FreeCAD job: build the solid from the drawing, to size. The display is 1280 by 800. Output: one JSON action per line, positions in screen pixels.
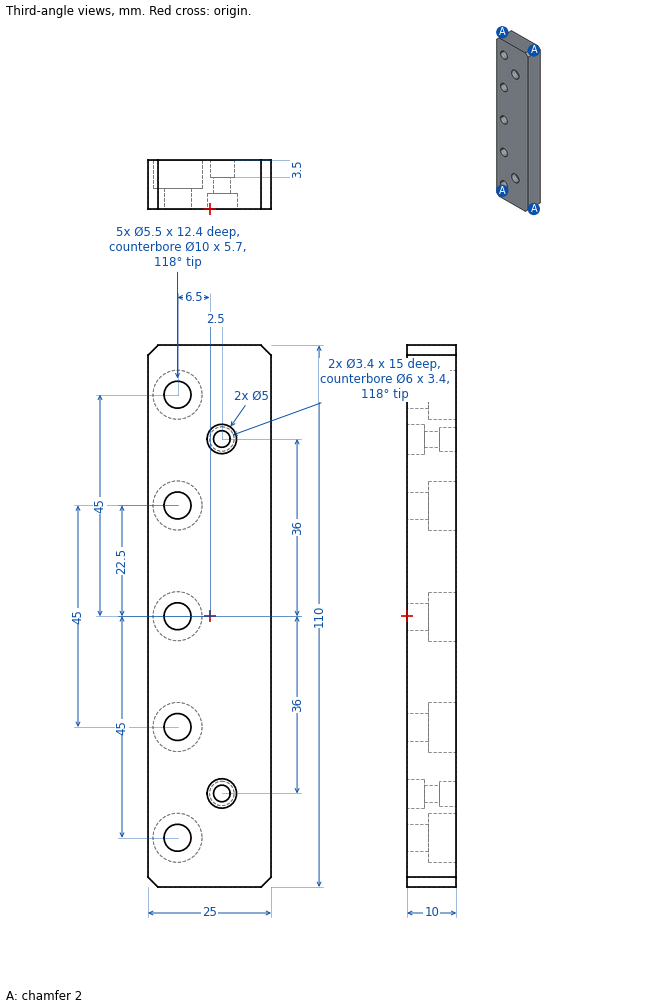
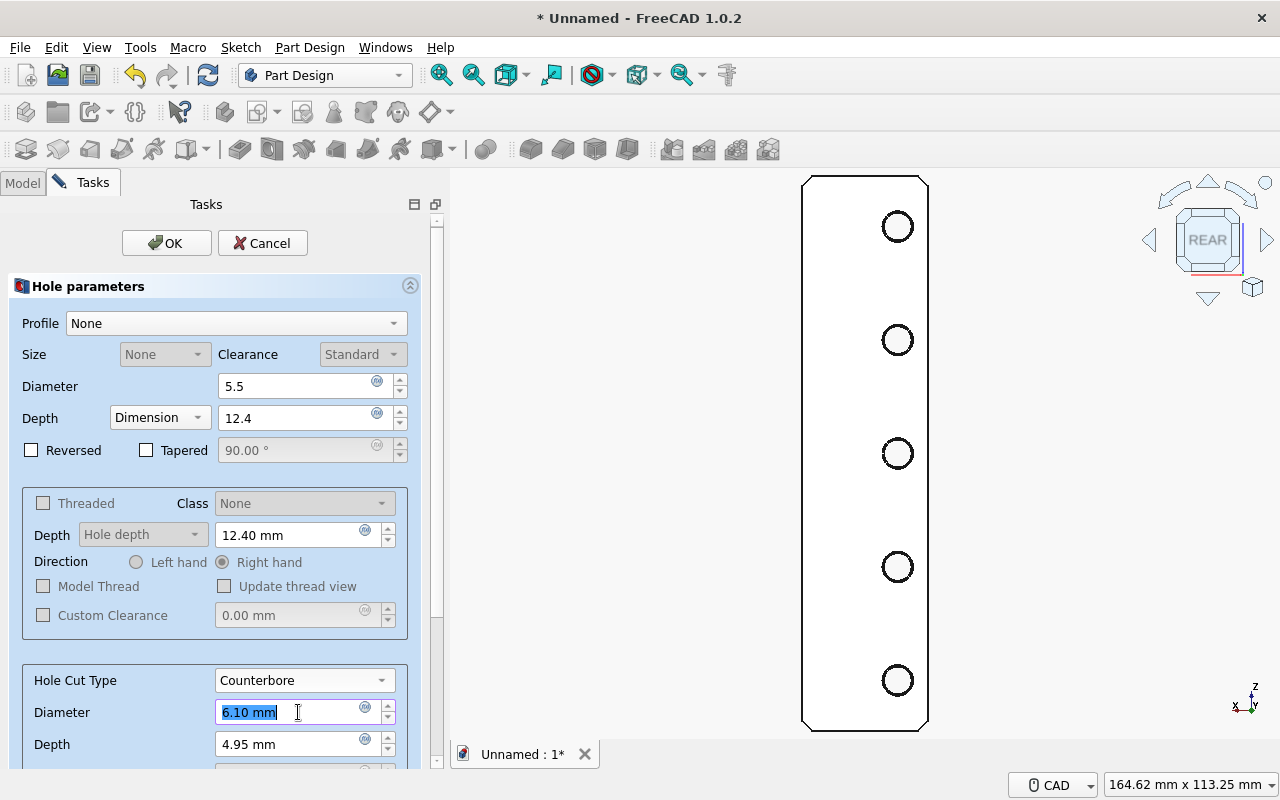
{"action": "type", "text": "10"}
{"action": "key", "text": "Tab"}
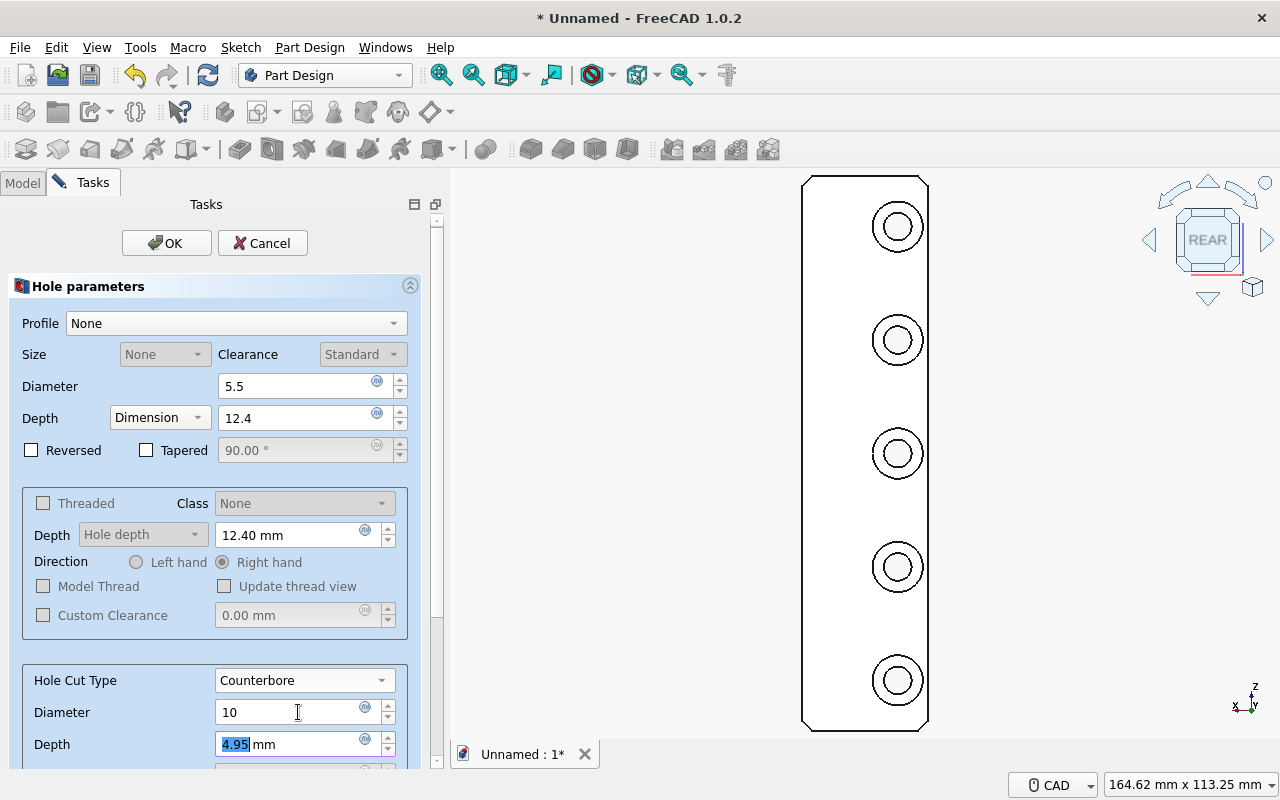
{"action": "type", "text": "5.7"}
{"action": "key", "text": "Tab"}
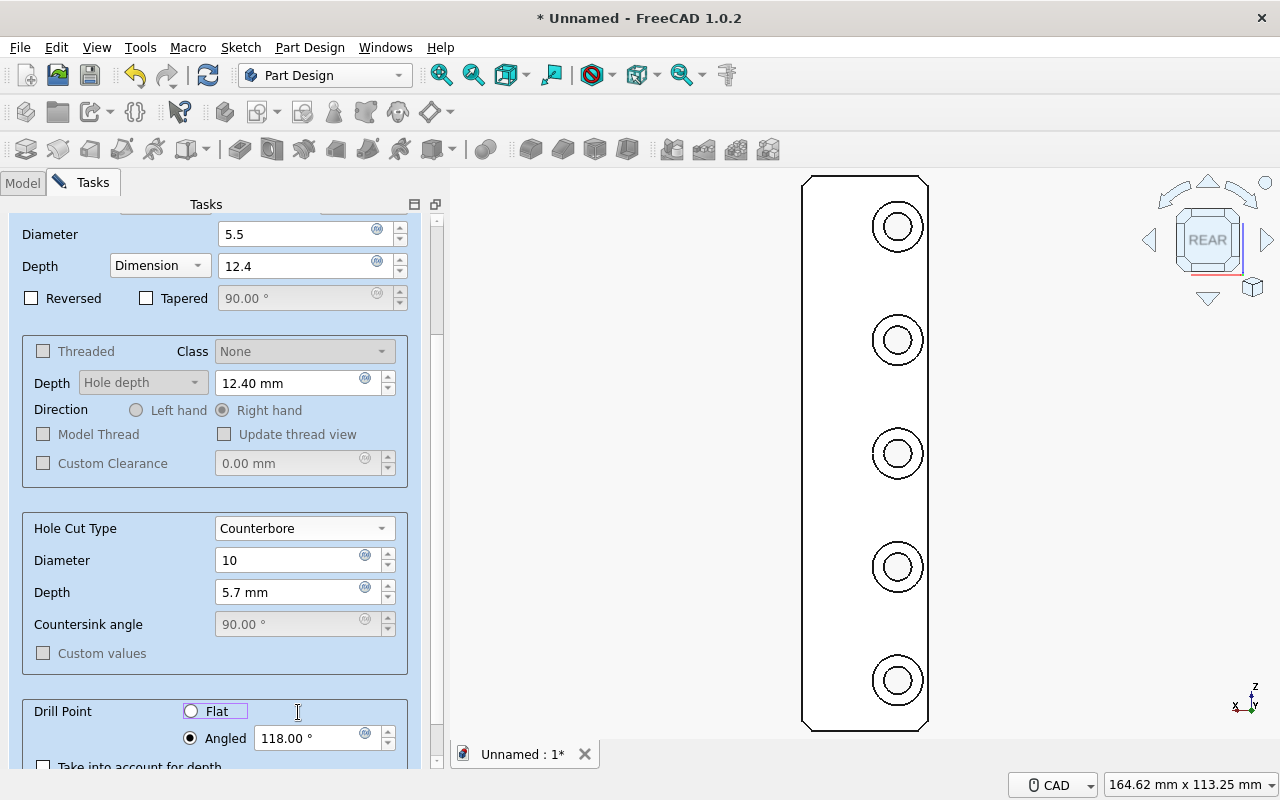
{"action": "scroll", "coordinate": [437, 491], "scroll_direction": "up", "scroll_amount": 4}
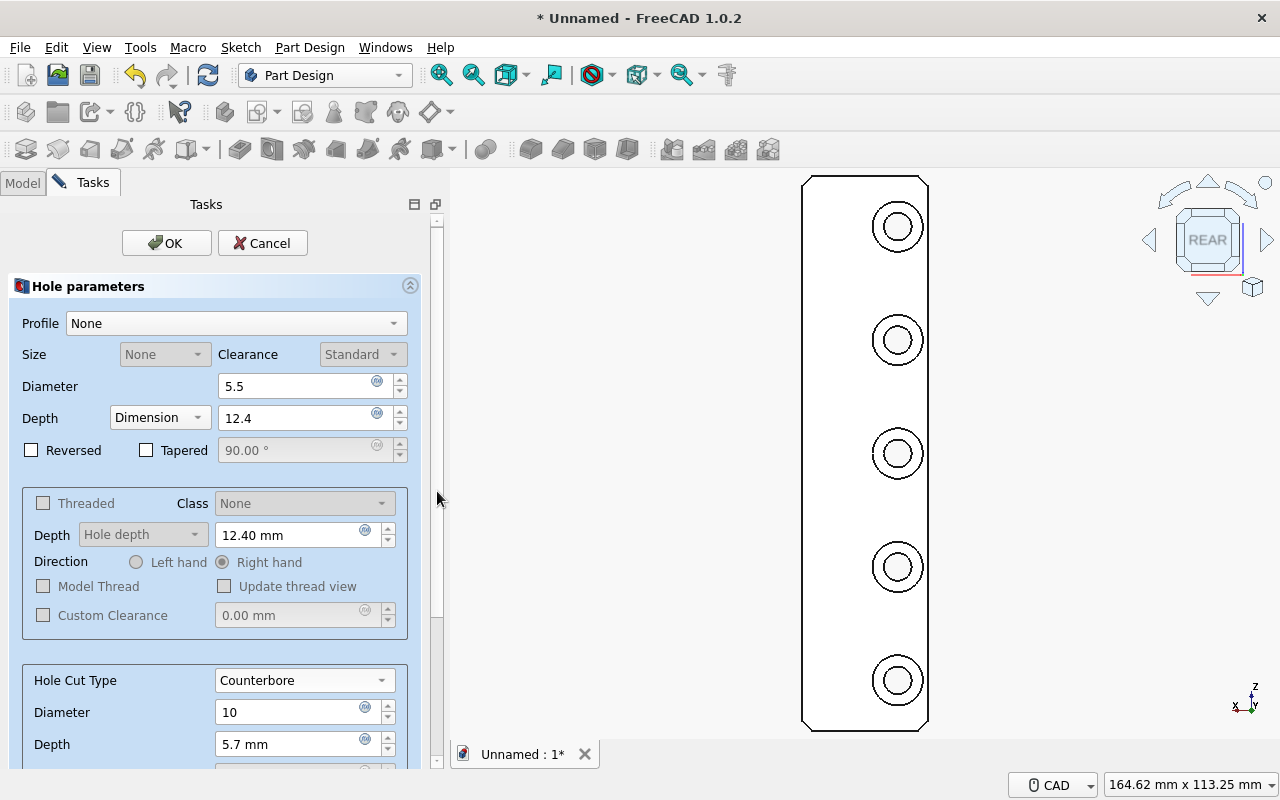
{"action": "left_click", "coordinate": [167, 243]}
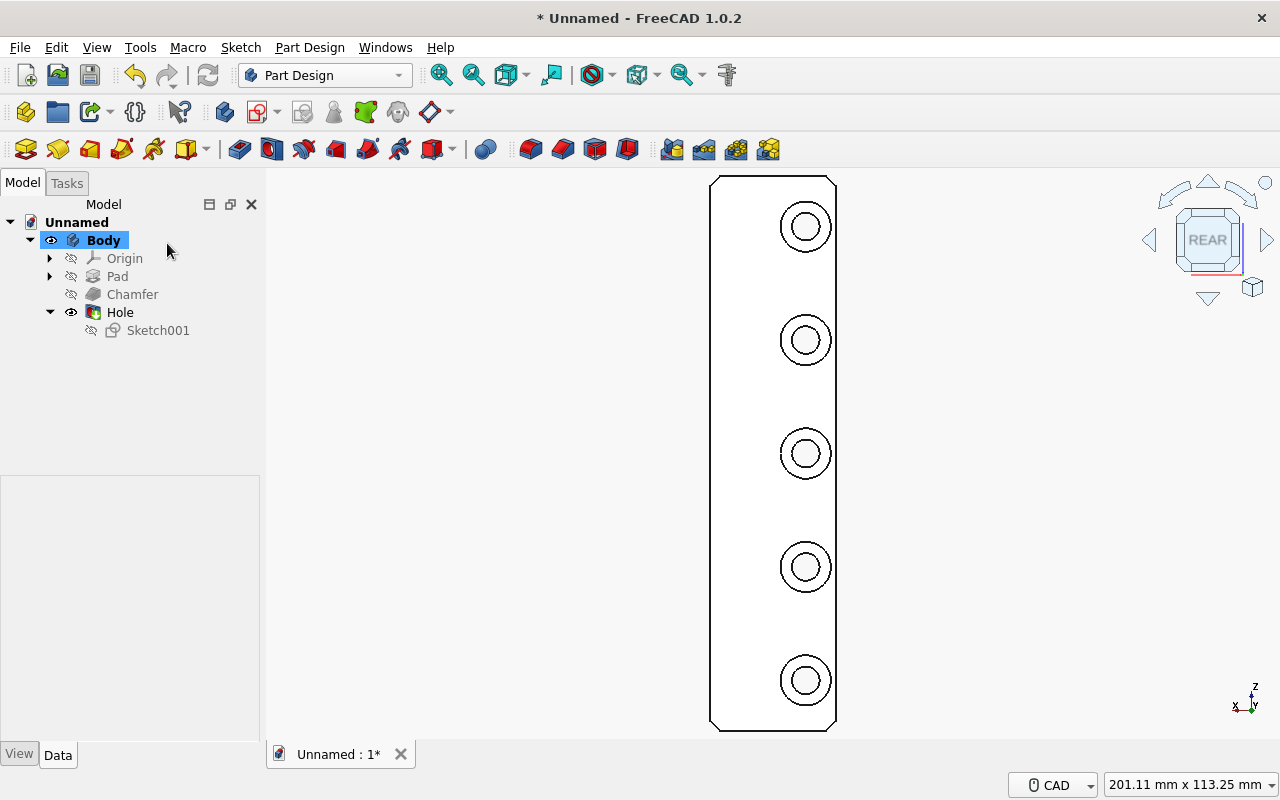
{"action": "left_click", "coordinate": [258, 112]}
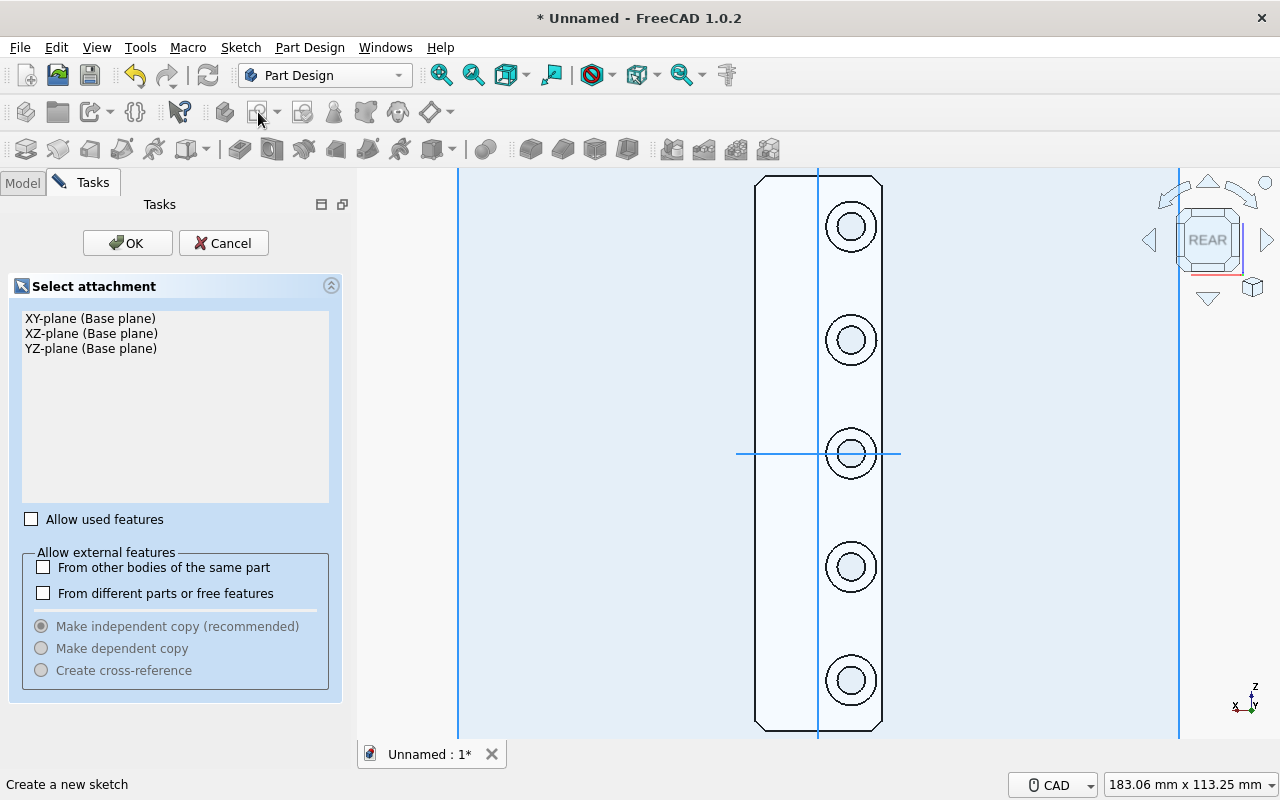
{"action": "left_click", "coordinate": [82, 334]}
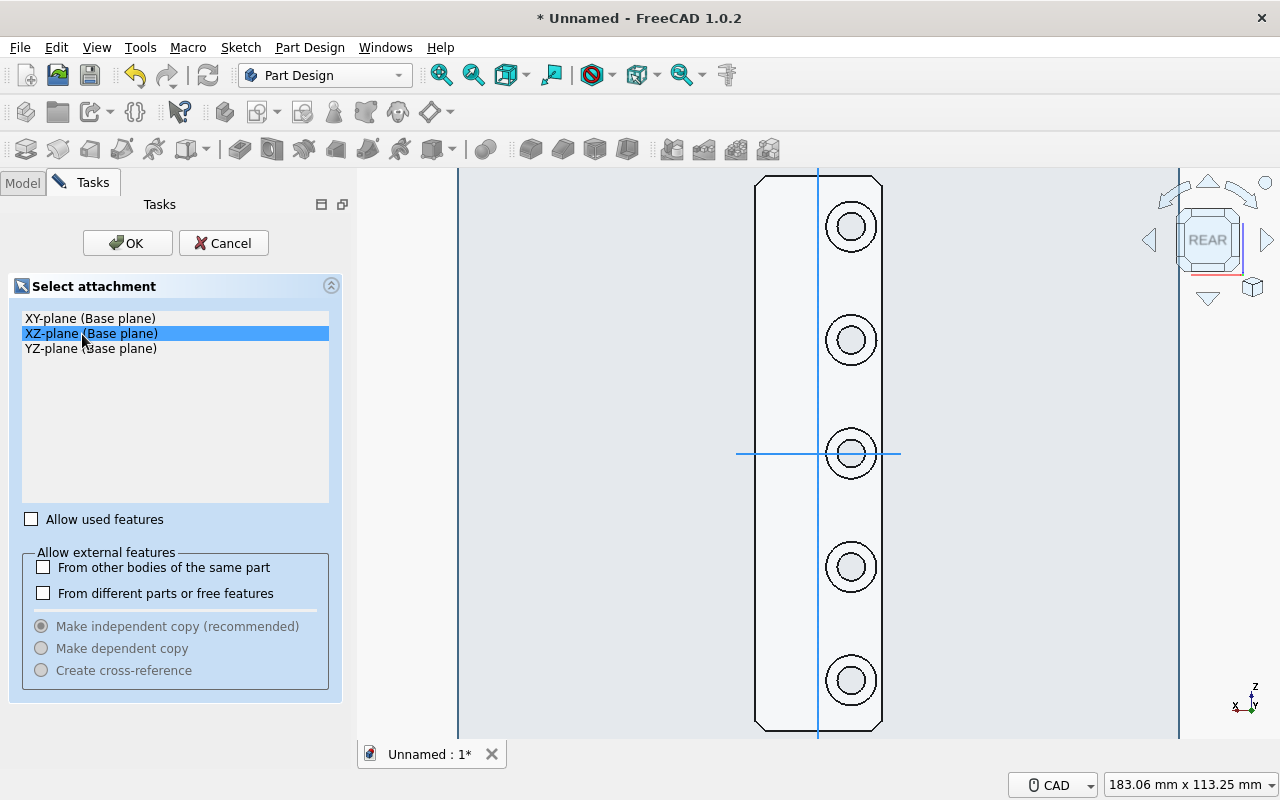
{"action": "left_click", "coordinate": [128, 243]}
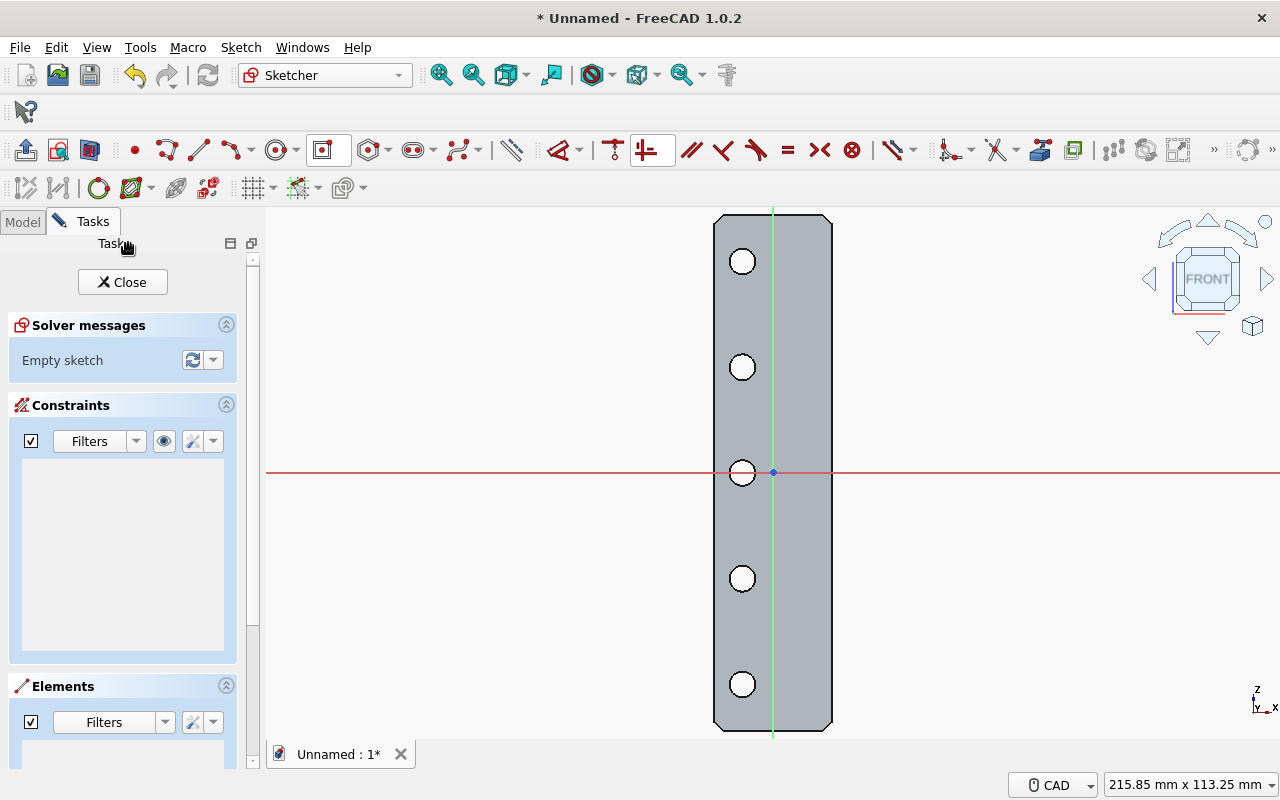
{"action": "left_click", "coordinate": [276, 150]}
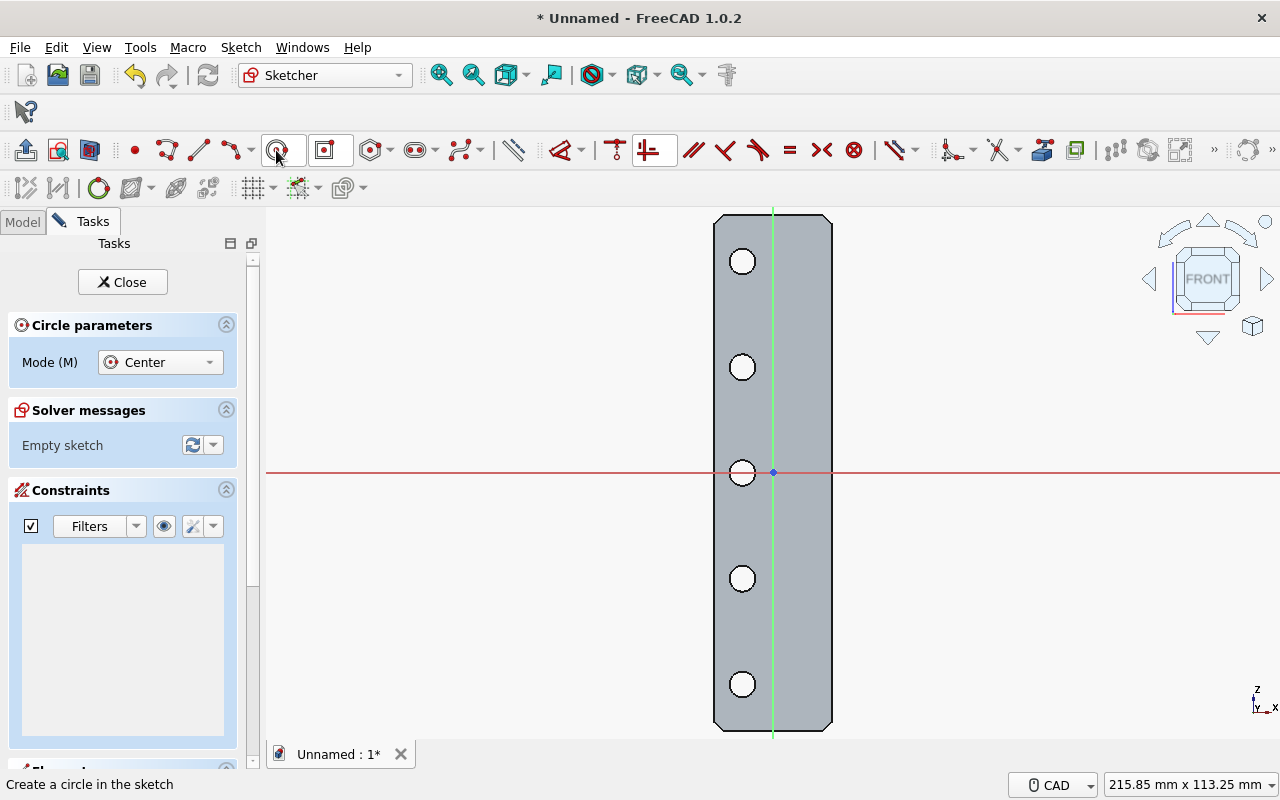
{"action": "scroll", "coordinate": [785, 304], "scroll_direction": "up", "scroll_amount": 6}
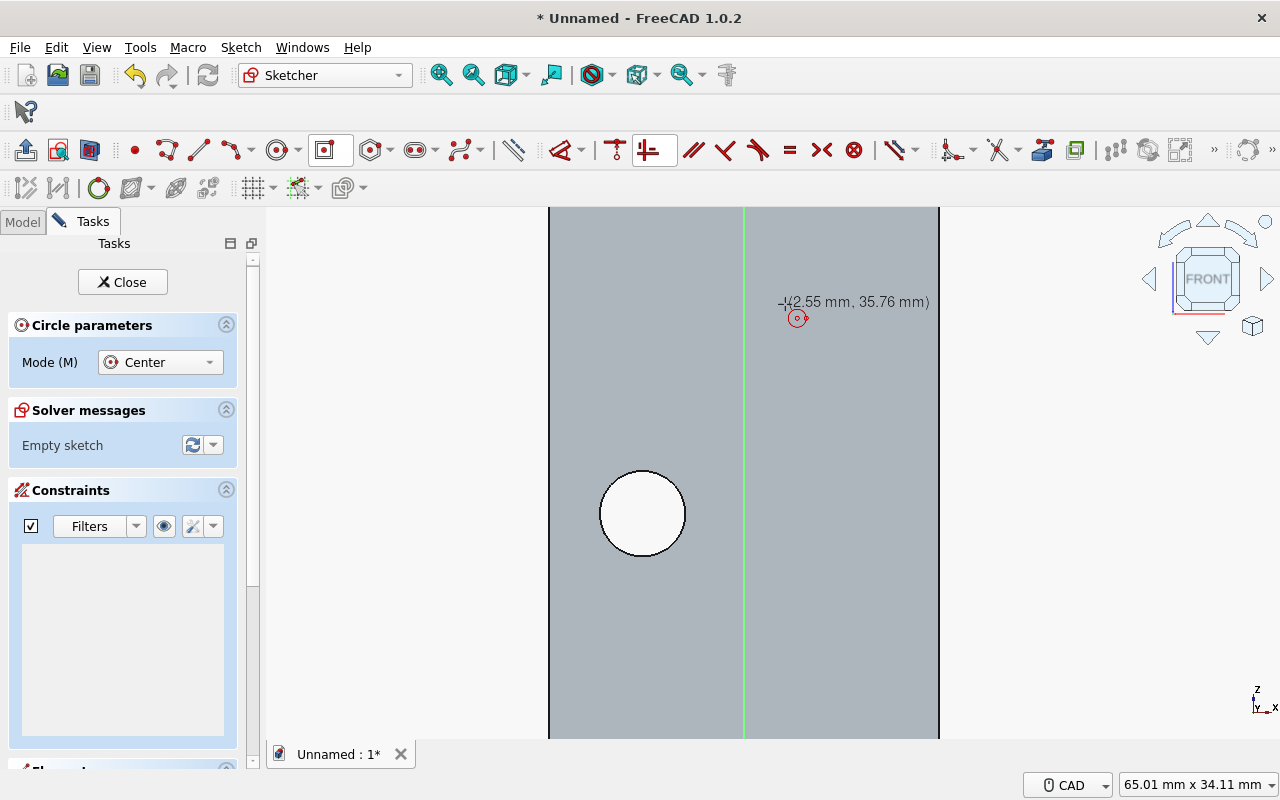
{"action": "left_click", "coordinate": [783, 303]}
{"action": "mouse_move", "coordinate": [802, 284]}